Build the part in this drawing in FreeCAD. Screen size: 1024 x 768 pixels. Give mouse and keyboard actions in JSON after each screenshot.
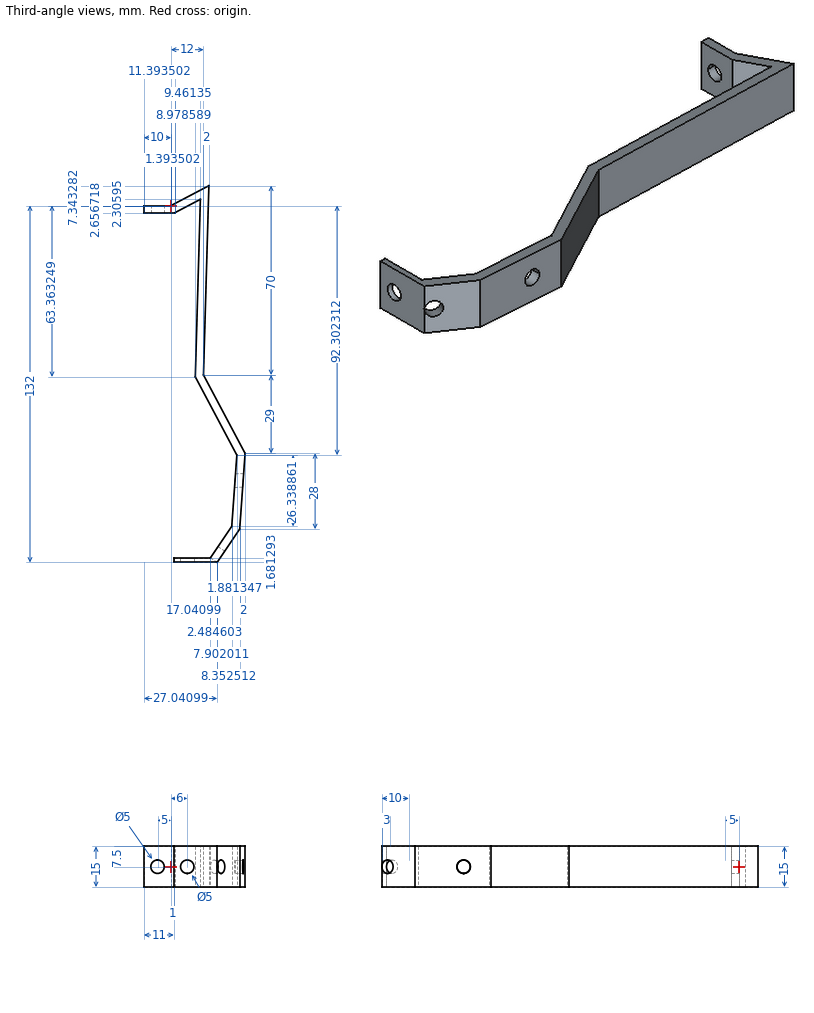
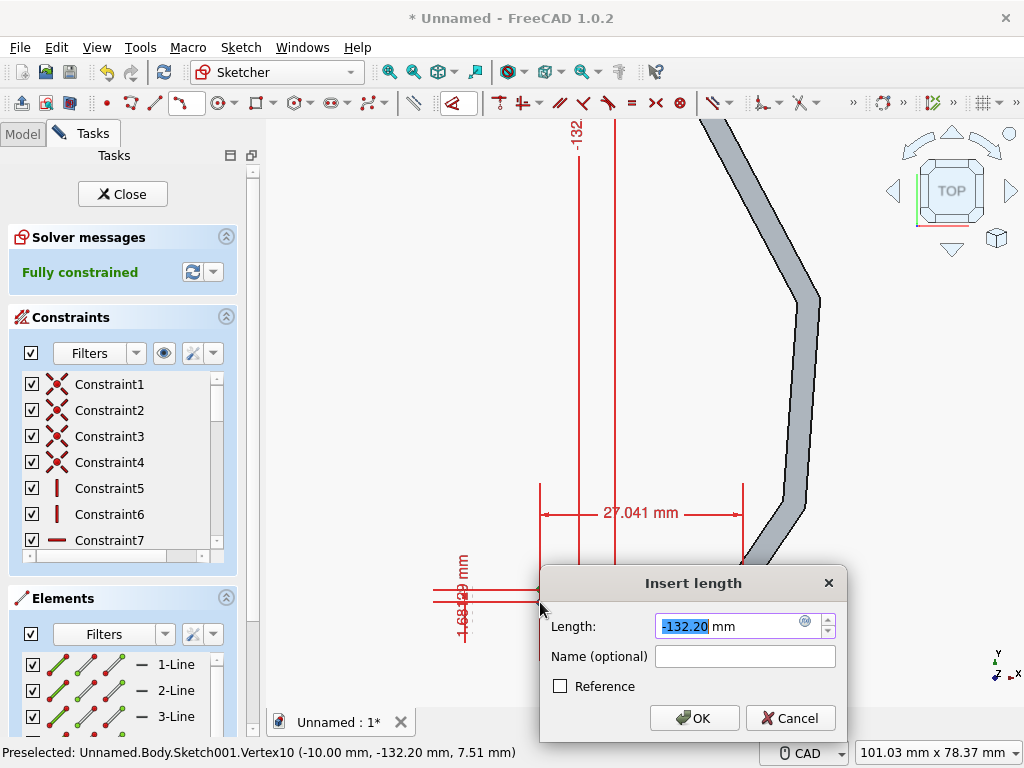
{"action": "type", "text": "-132"}
{"action": "key", "text": "Return"}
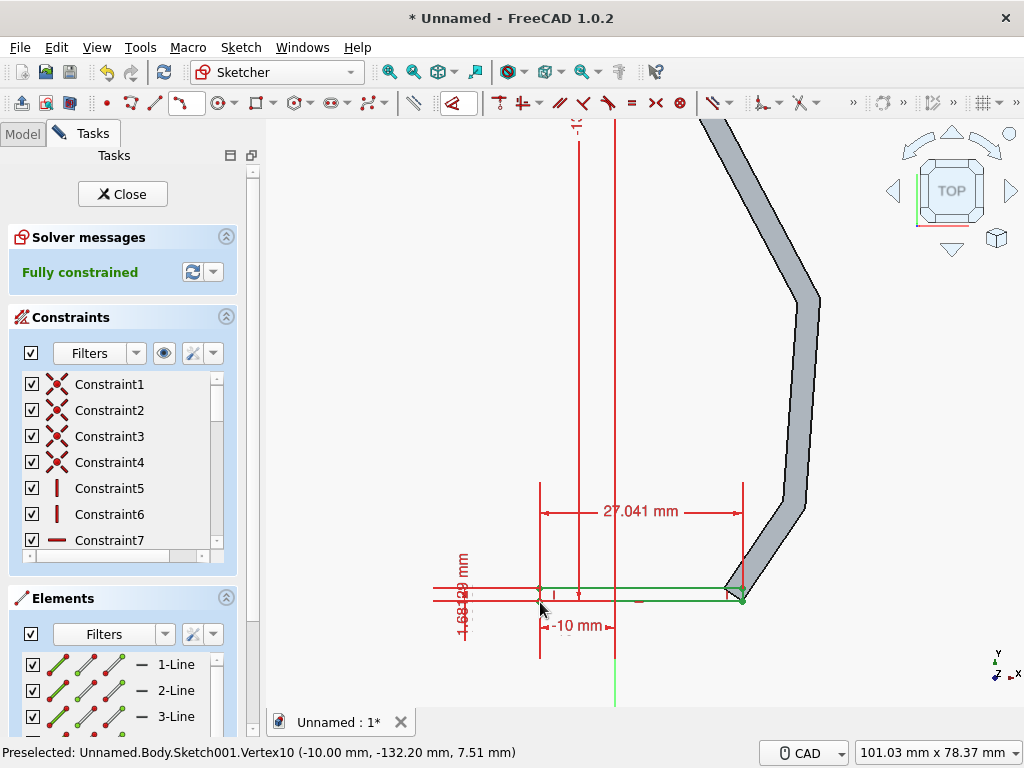
{"action": "left_click", "coordinate": [123, 194]}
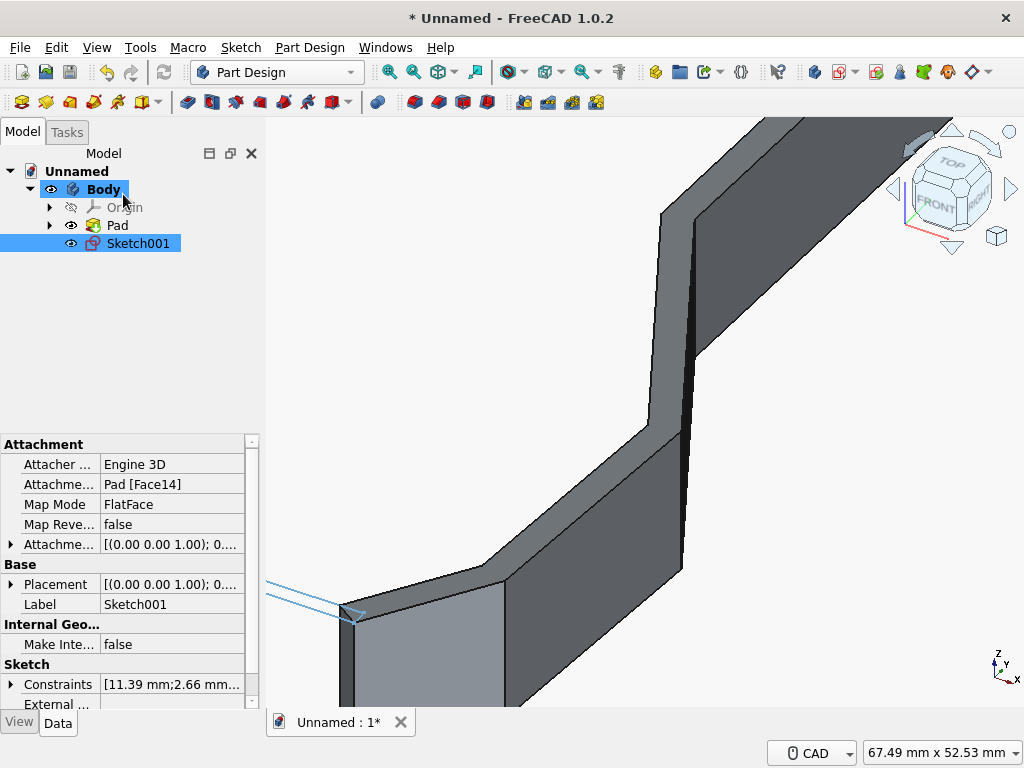
{"action": "left_click", "coordinate": [22, 102]}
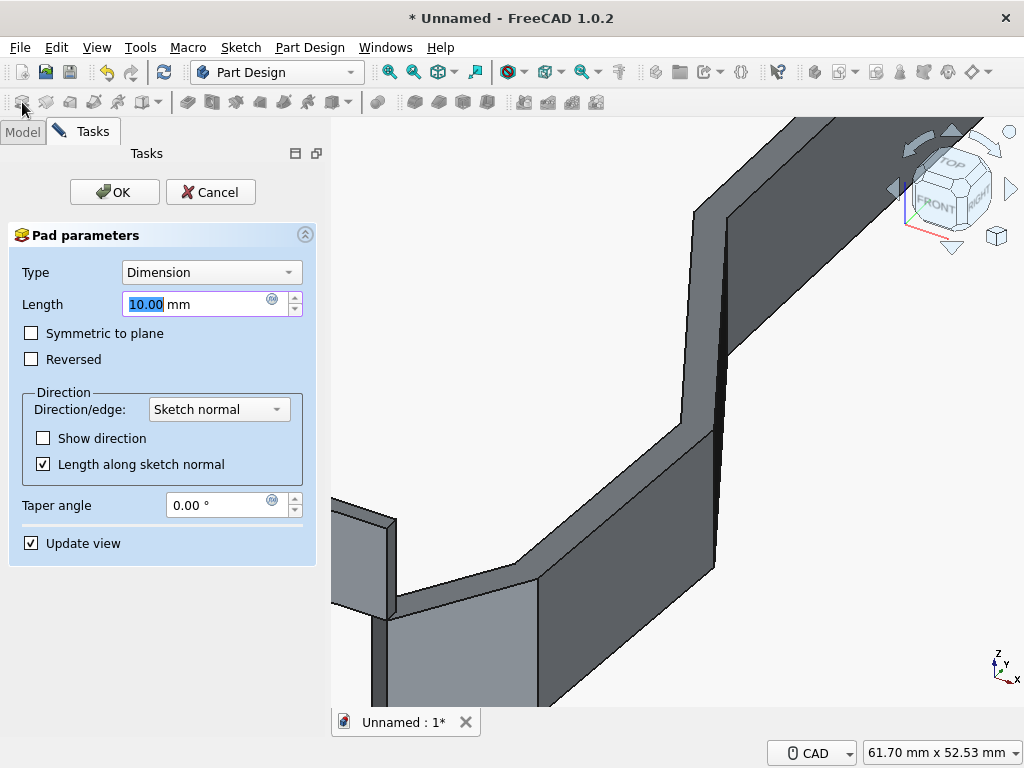
{"action": "type", "text": "15"}
{"action": "key", "text": "Tab"}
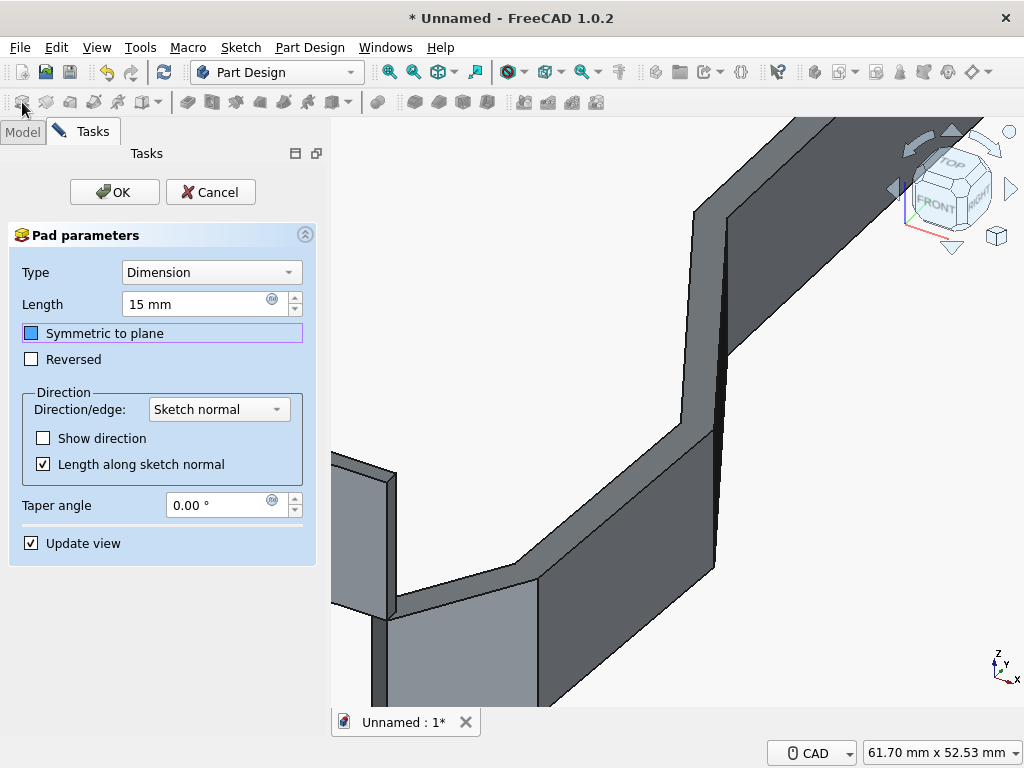
{"action": "left_click", "coordinate": [30, 359]}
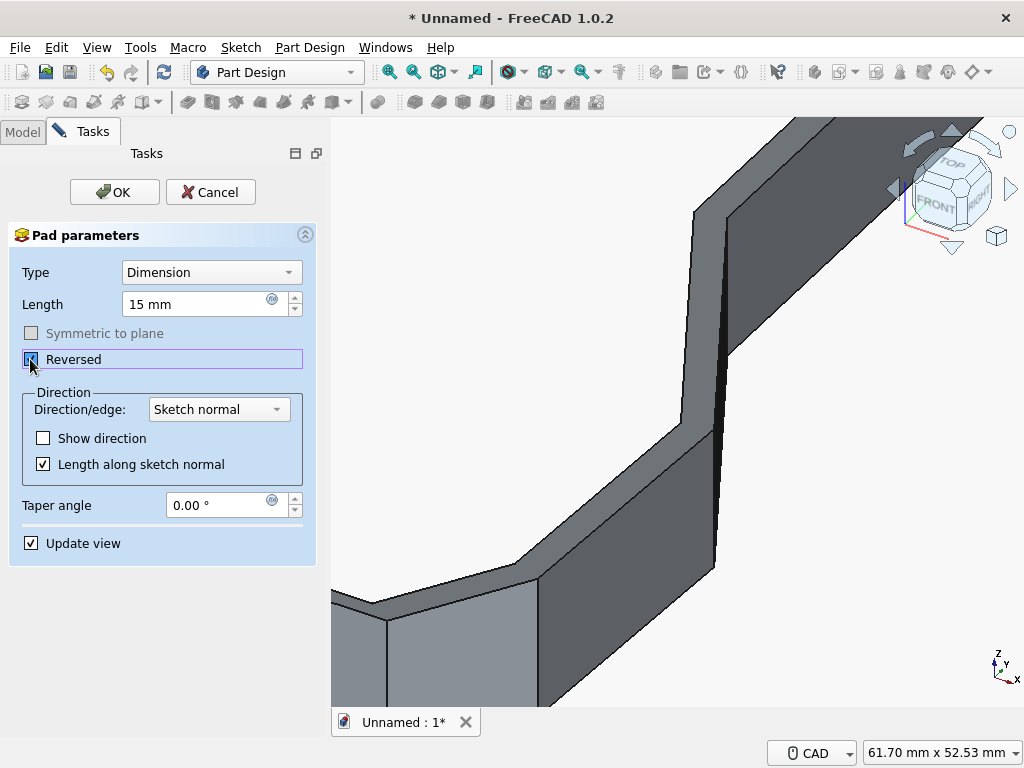
{"action": "left_click", "coordinate": [115, 192]}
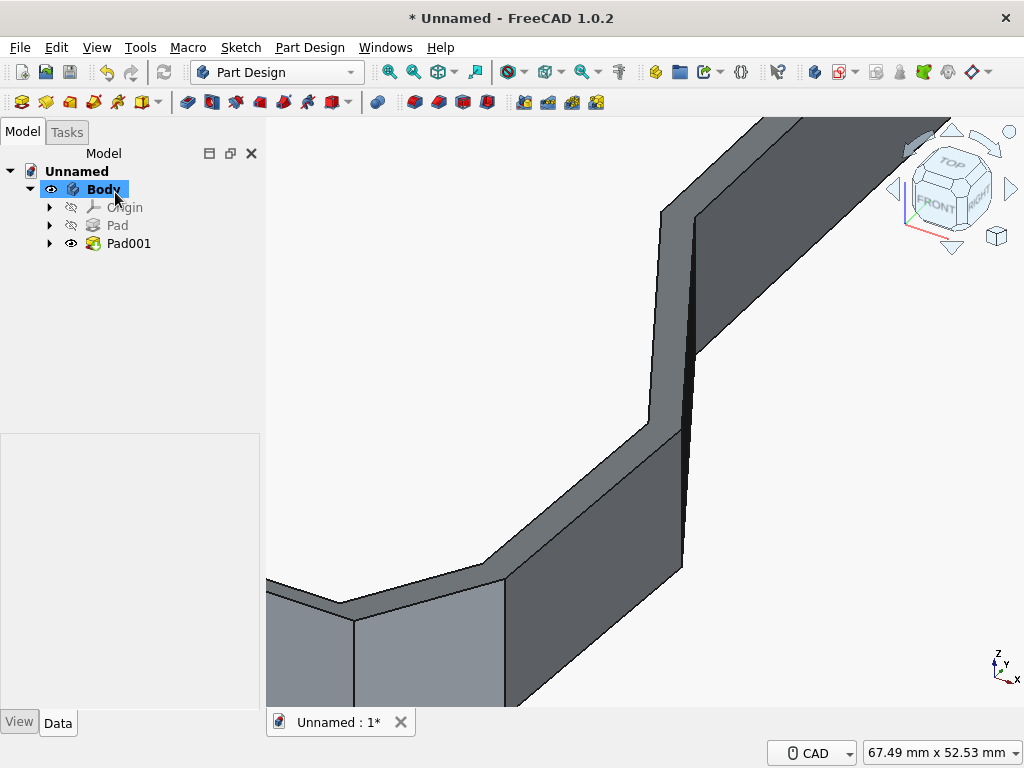
{"action": "left_click", "coordinate": [390, 72]}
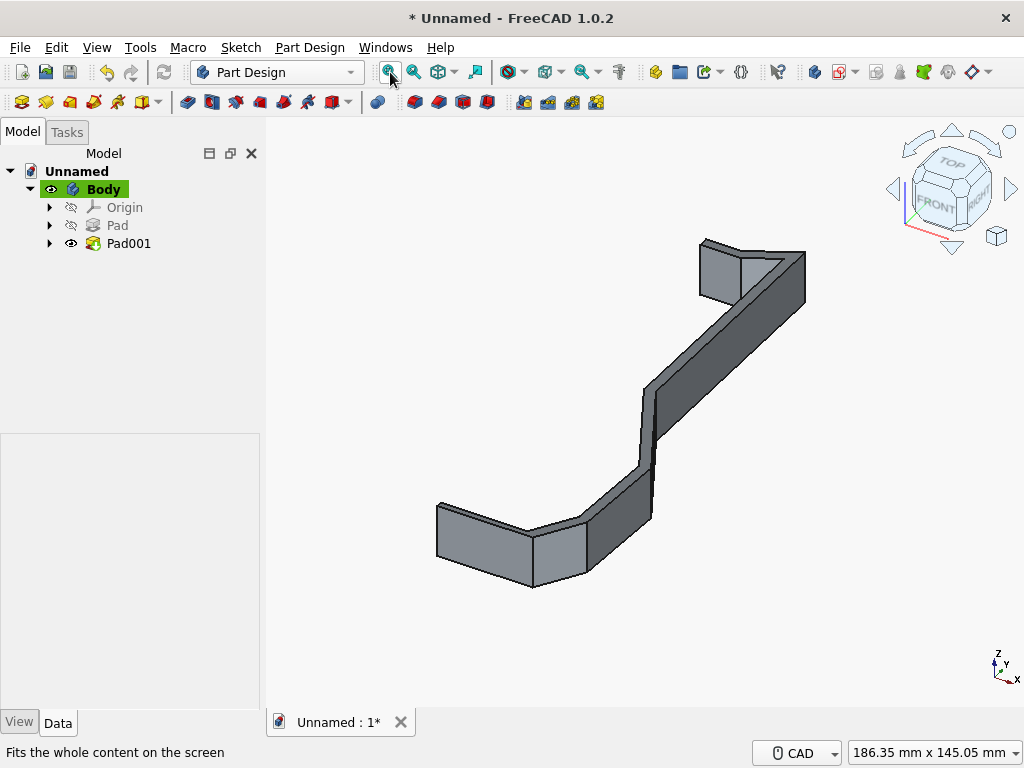
{"action": "key", "text": "4"}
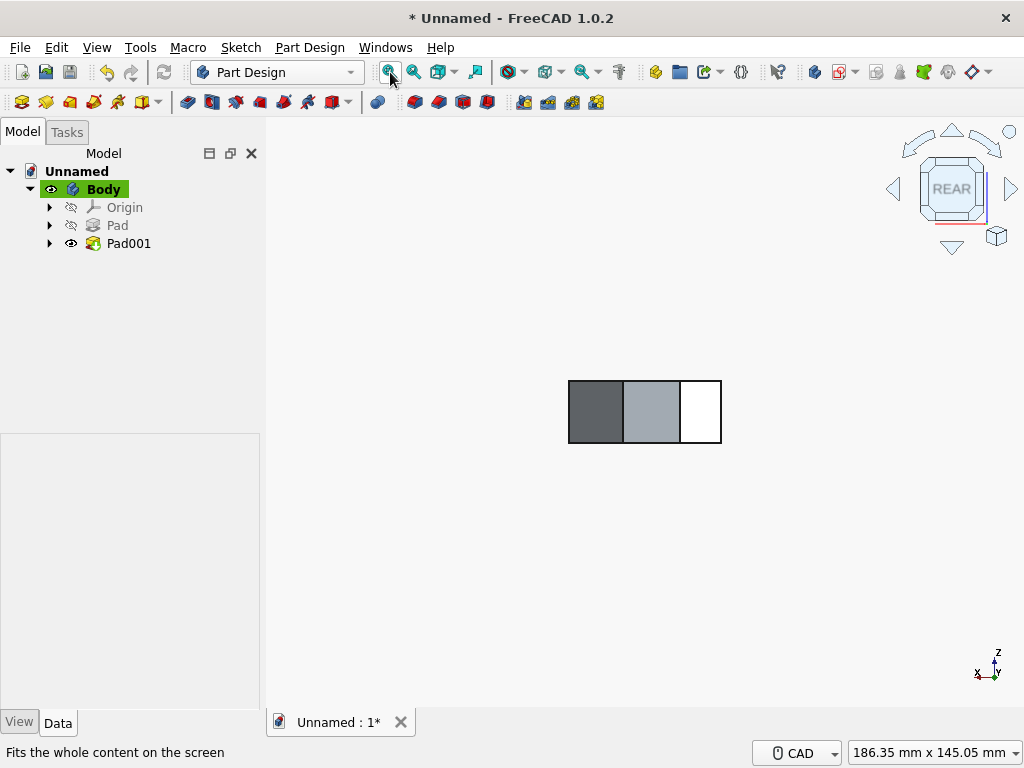
{"action": "left_click", "coordinate": [390, 72]}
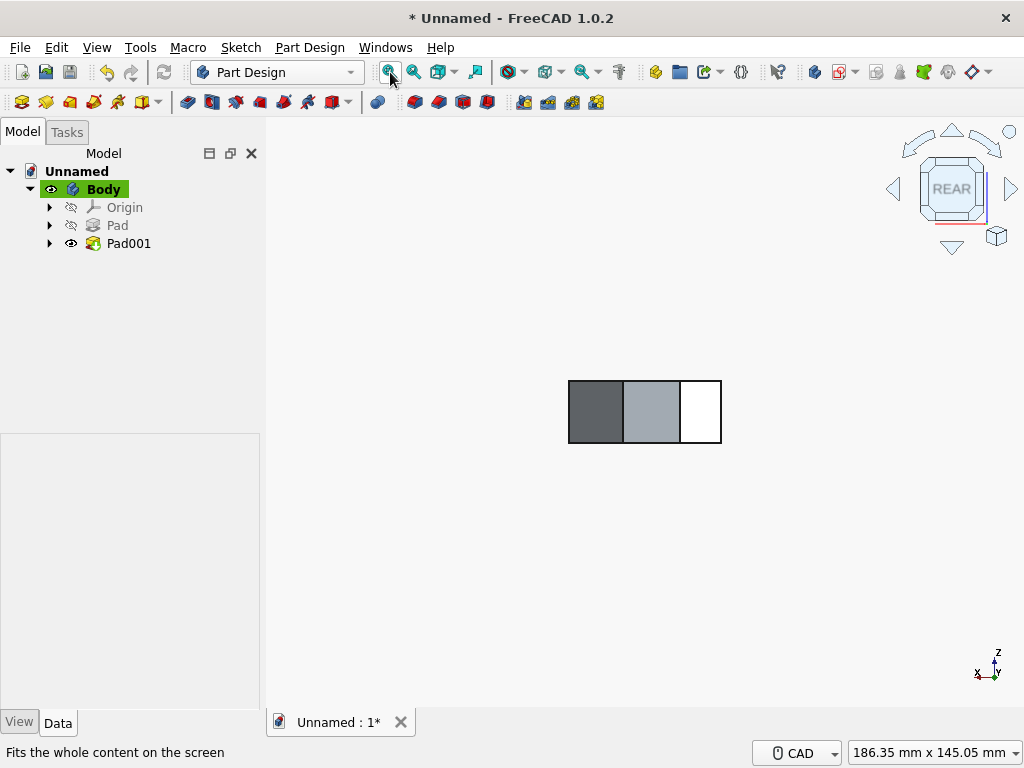
{"action": "left_click", "coordinate": [701, 402]}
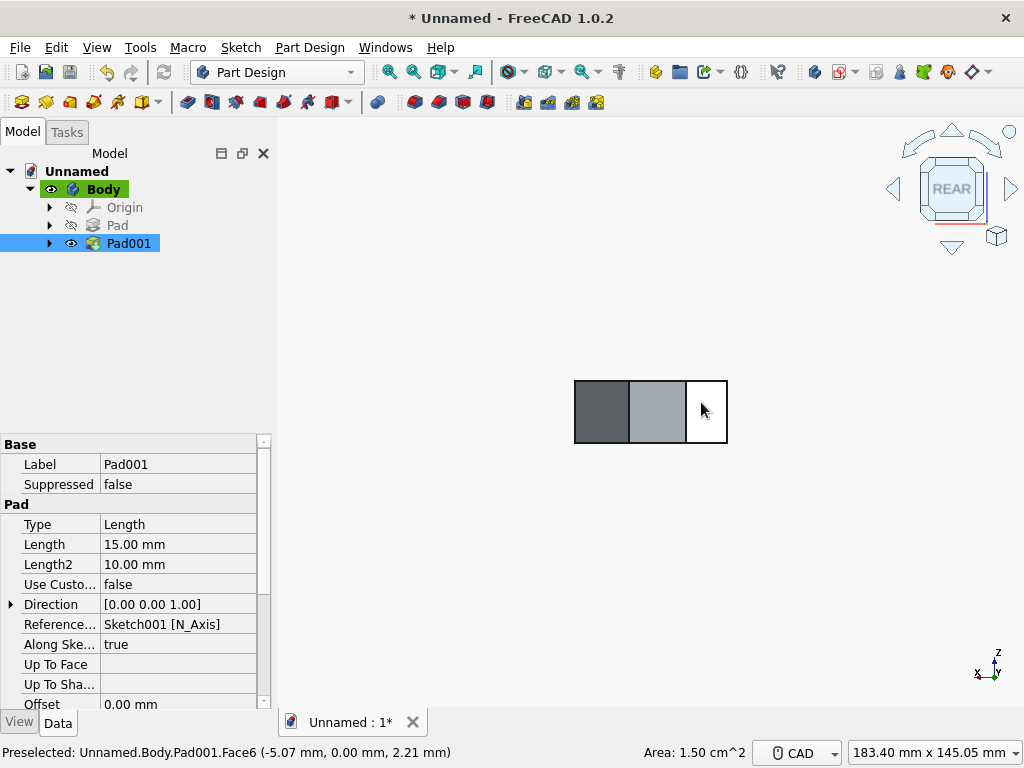
{"action": "left_click", "coordinate": [840, 72]}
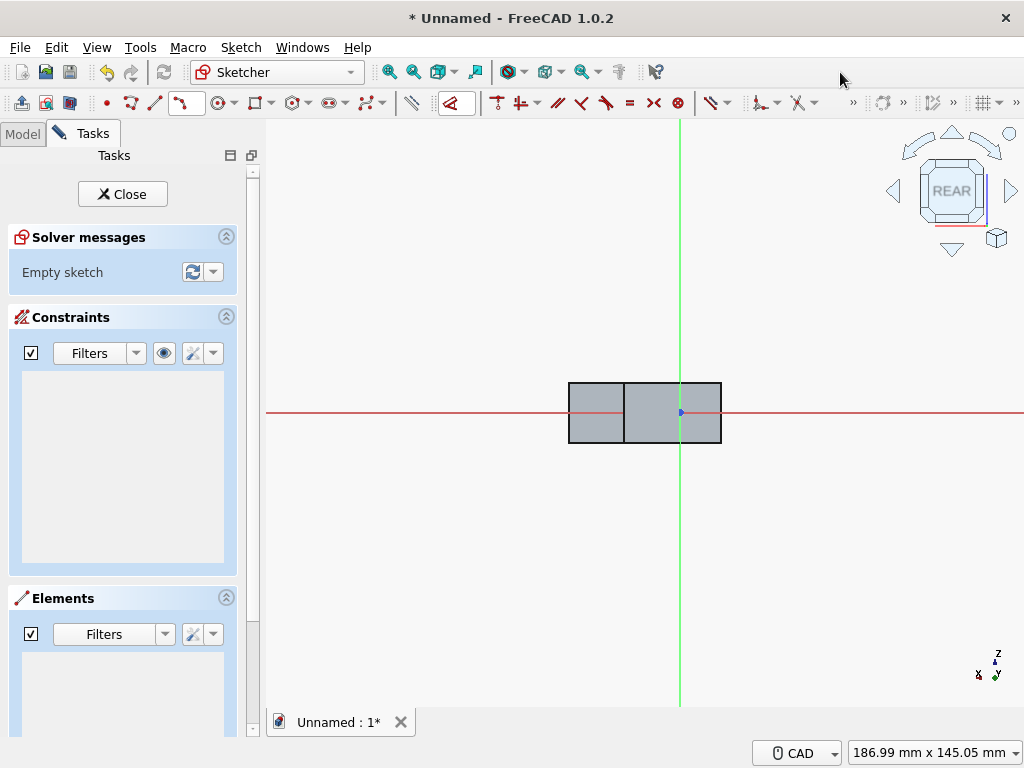
{"action": "left_click", "coordinate": [70, 104]}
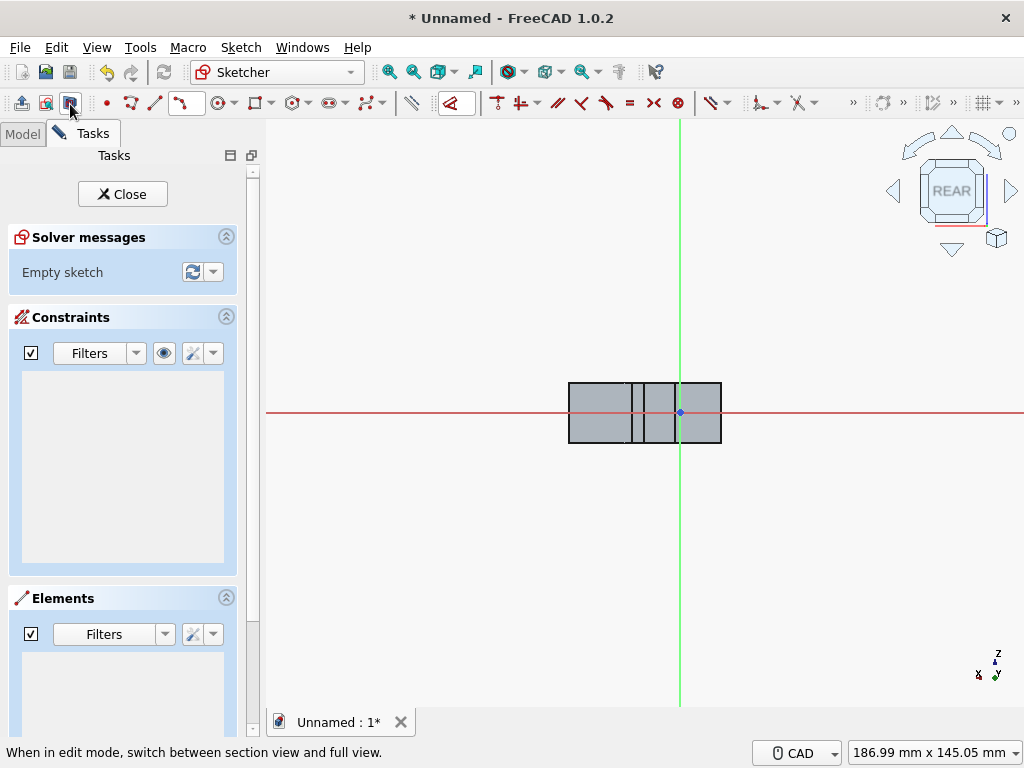
{"action": "scroll", "coordinate": [705, 413], "scroll_direction": "up", "scroll_amount": 13}